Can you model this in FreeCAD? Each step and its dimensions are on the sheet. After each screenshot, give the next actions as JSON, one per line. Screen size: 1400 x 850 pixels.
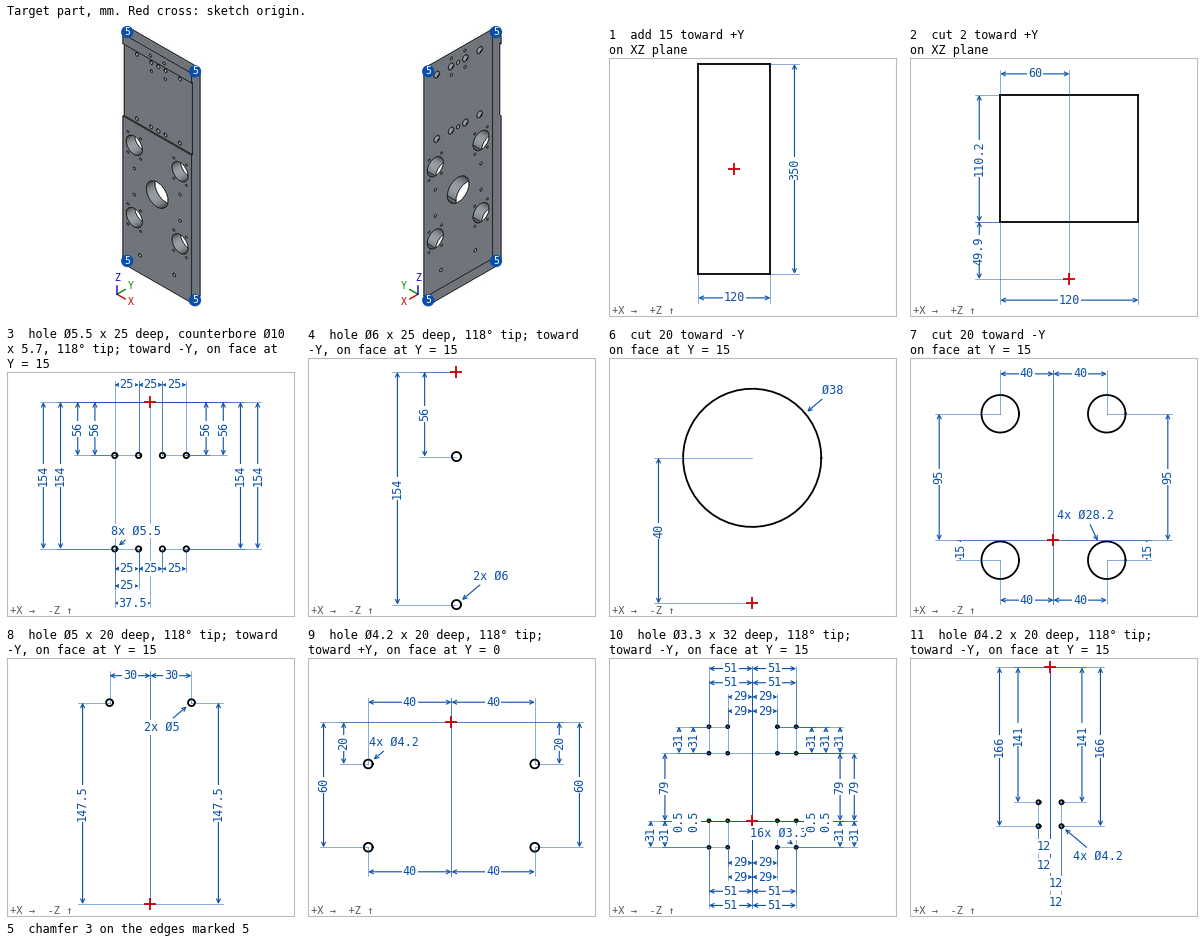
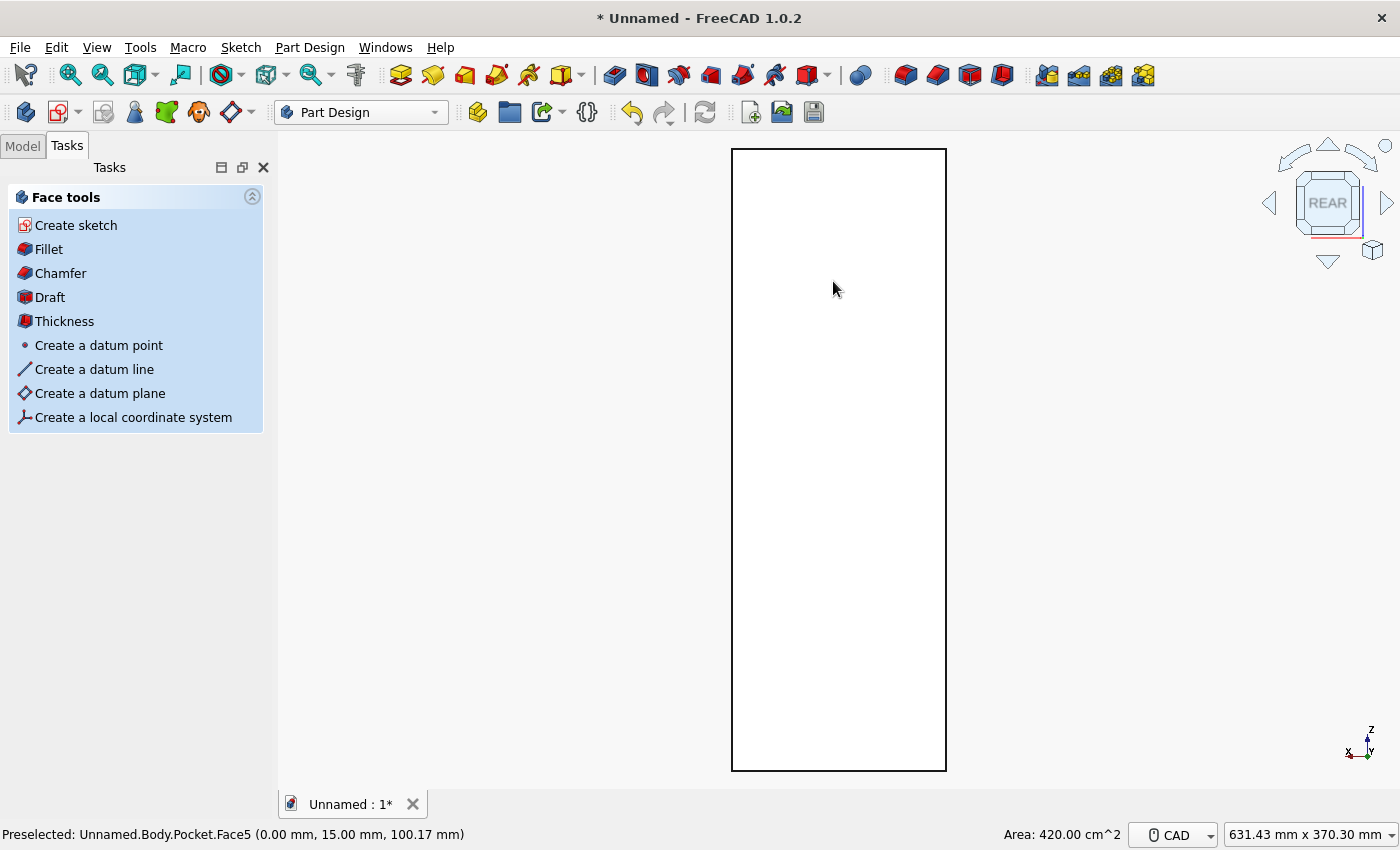
{"action": "left_click", "coordinate": [58, 112]}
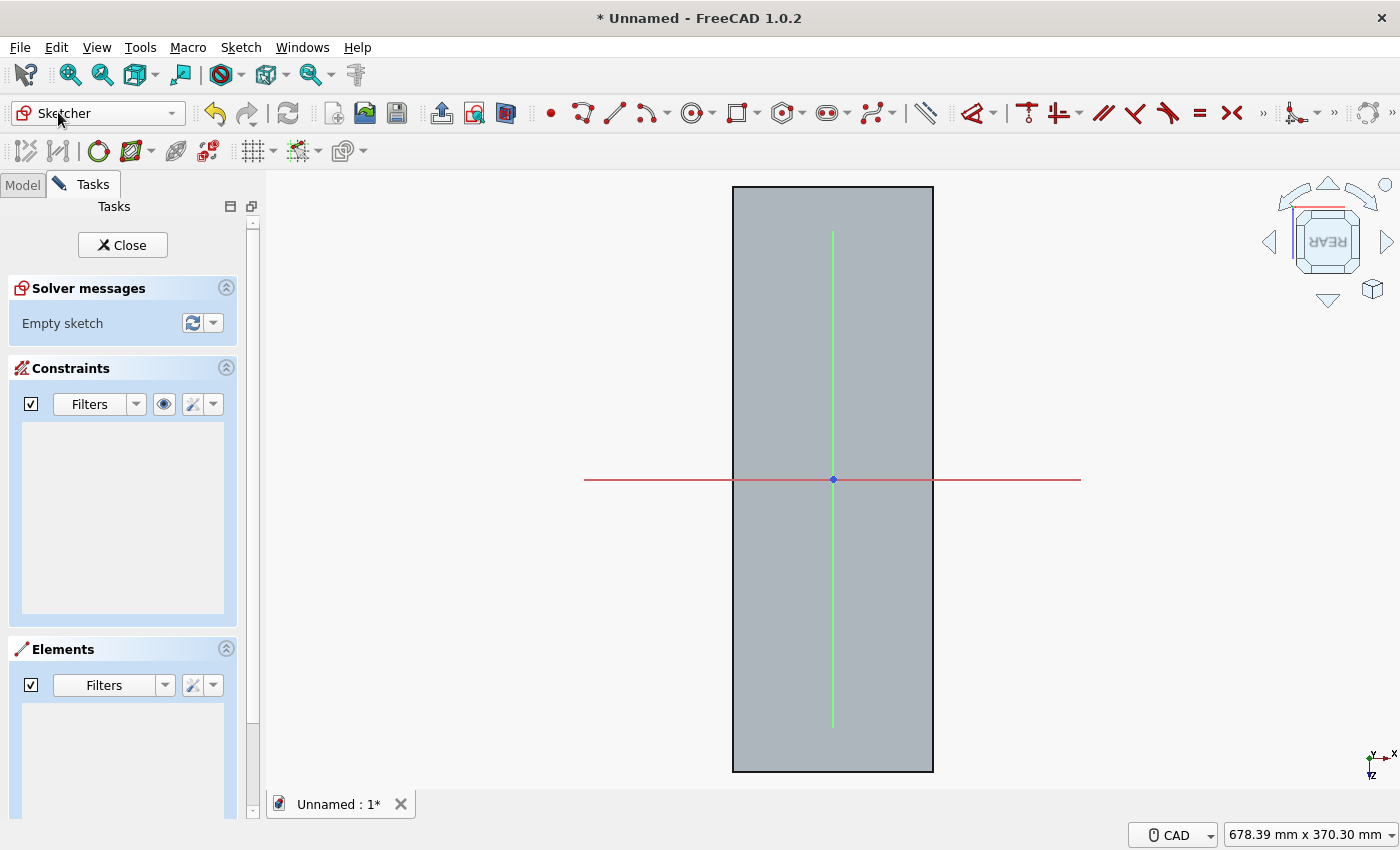
{"action": "scroll", "coordinate": [972, 761], "scroll_direction": "up", "scroll_amount": 2}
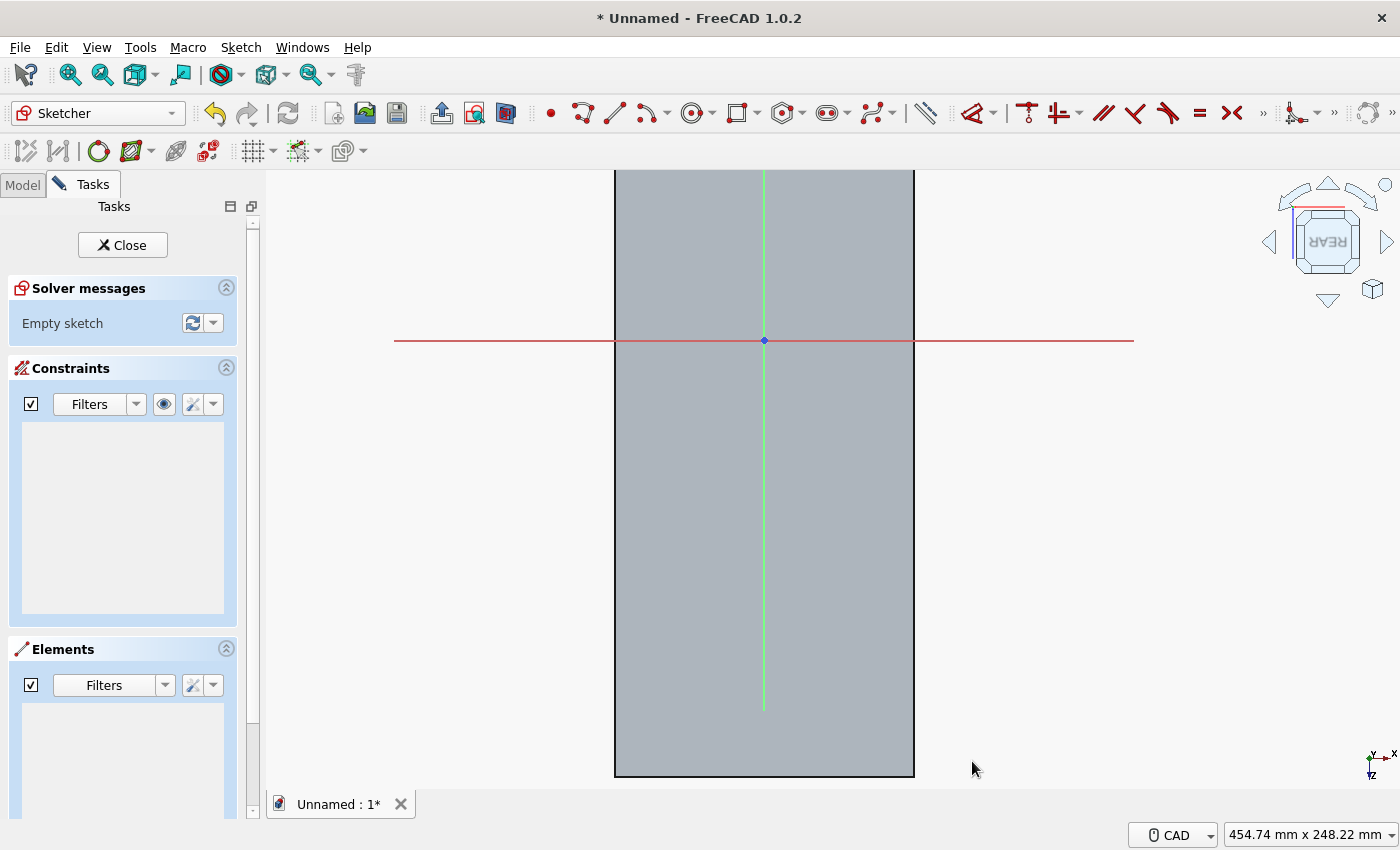
{"action": "left_click", "coordinate": [692, 114]}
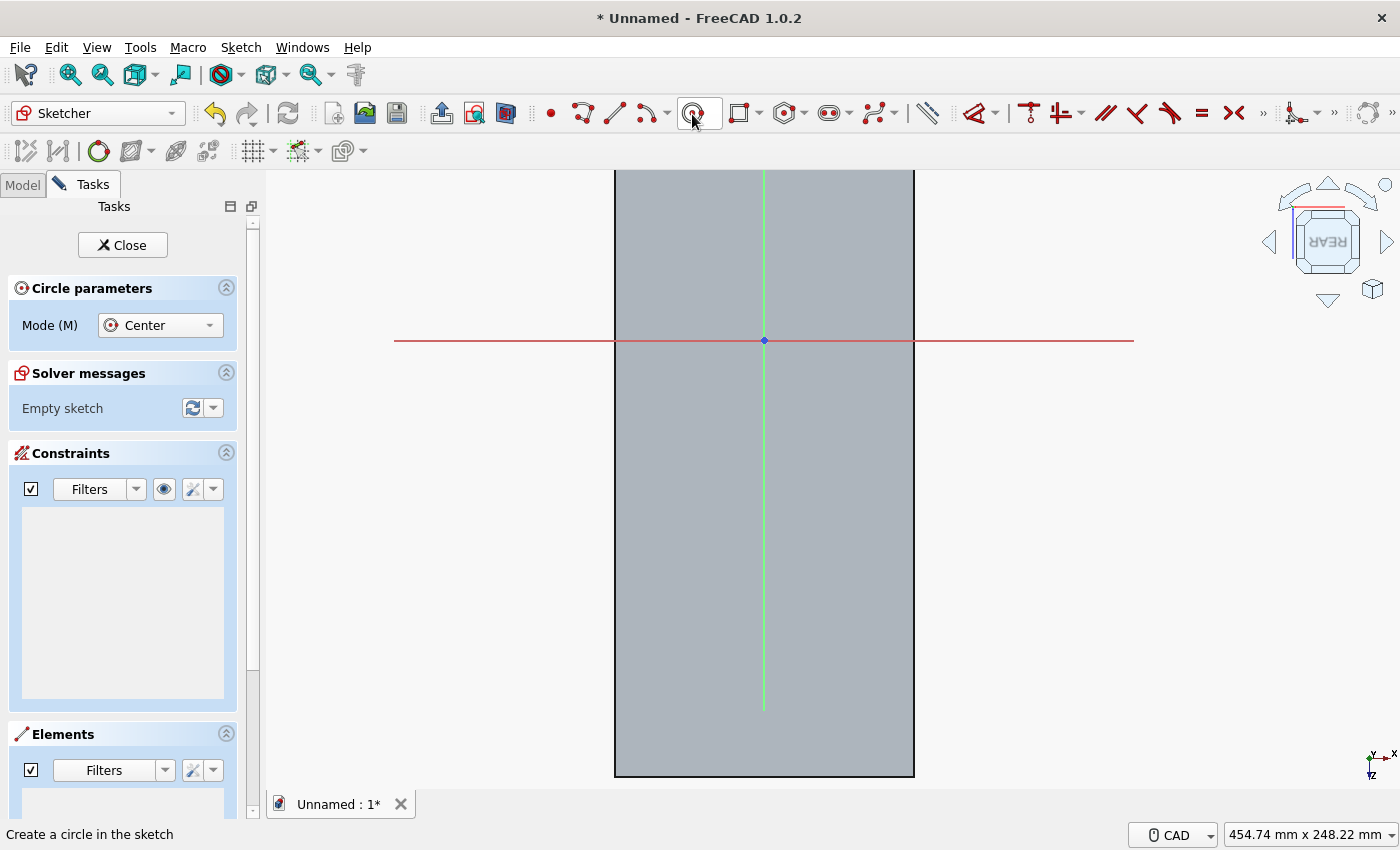
{"action": "scroll", "coordinate": [671, 725], "scroll_direction": "up", "scroll_amount": 6}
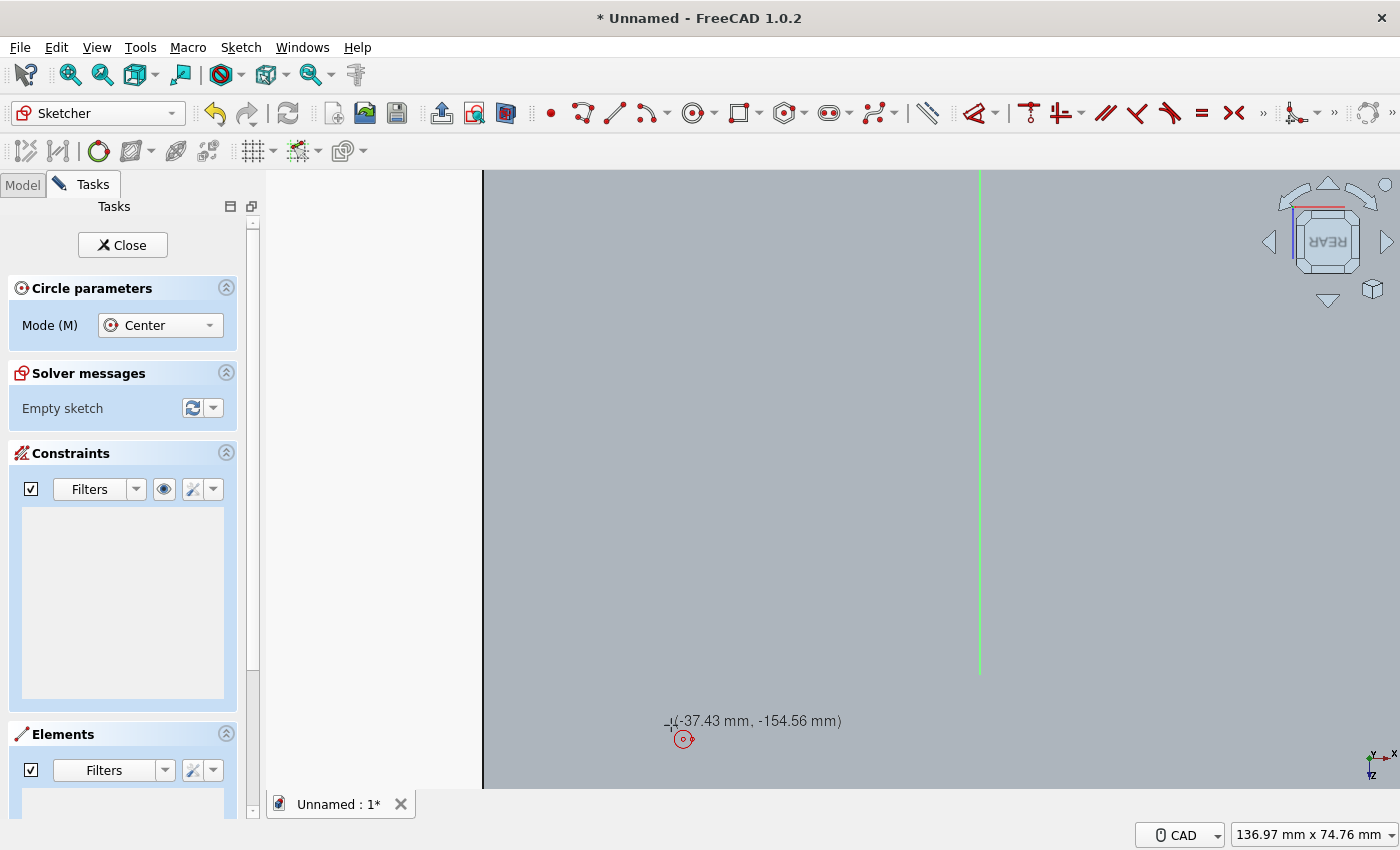
{"action": "left_click", "coordinate": [670, 722]}
{"action": "left_click", "coordinate": [686, 706]}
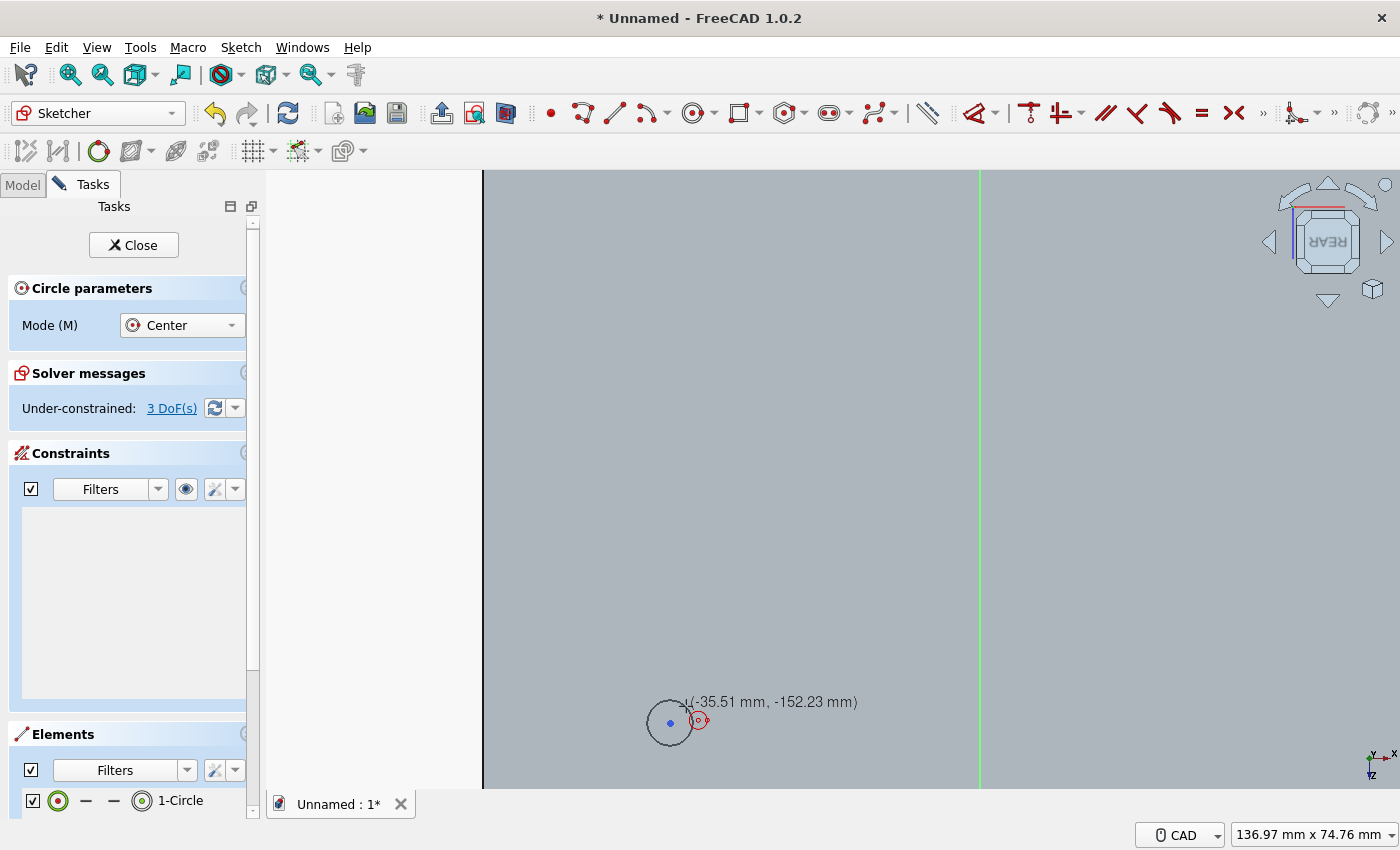
{"action": "left_click", "coordinate": [877, 722]}
{"action": "left_click", "coordinate": [893, 706]}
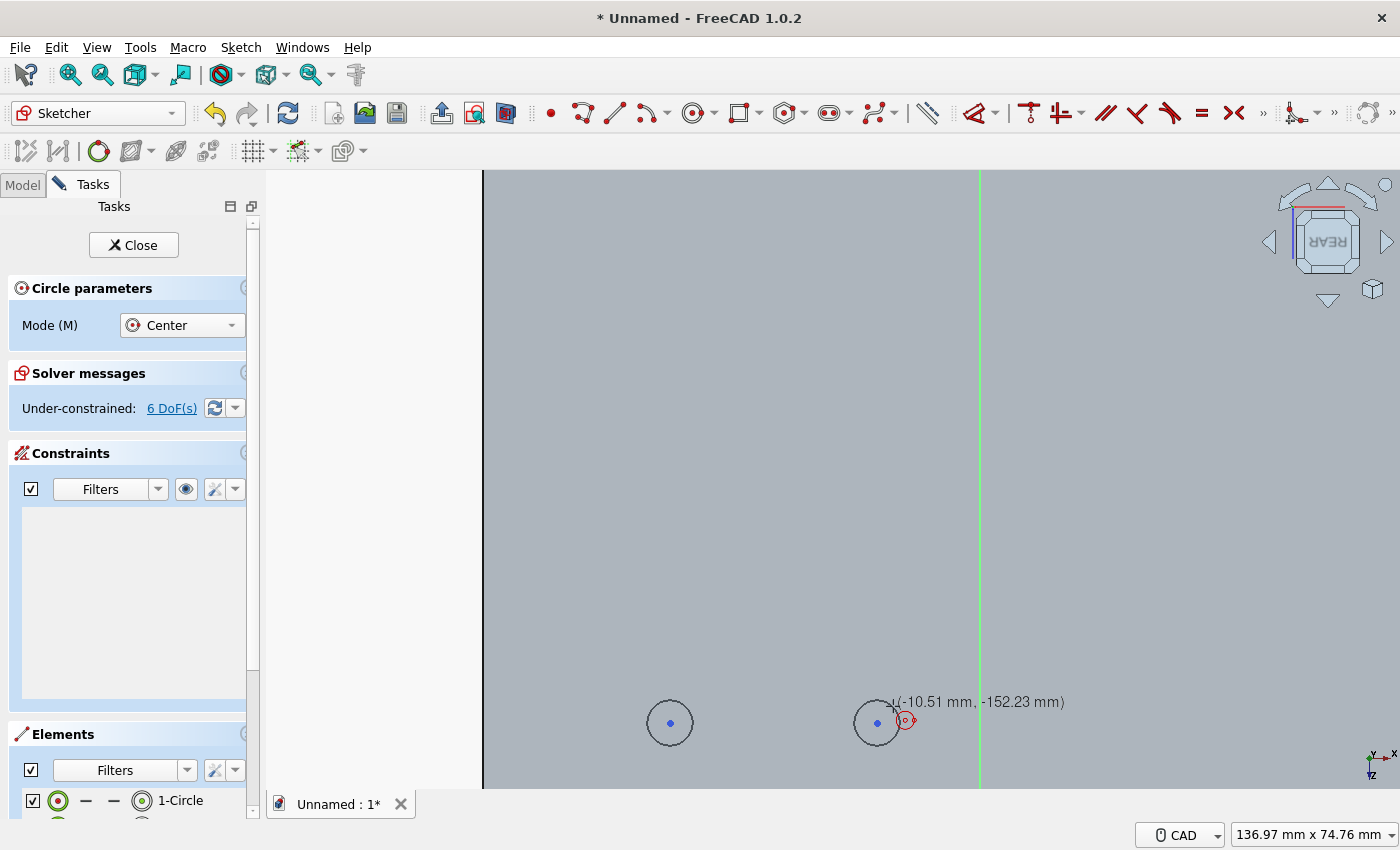
{"action": "left_click", "coordinate": [1084, 722]}
{"action": "left_click", "coordinate": [1100, 706]}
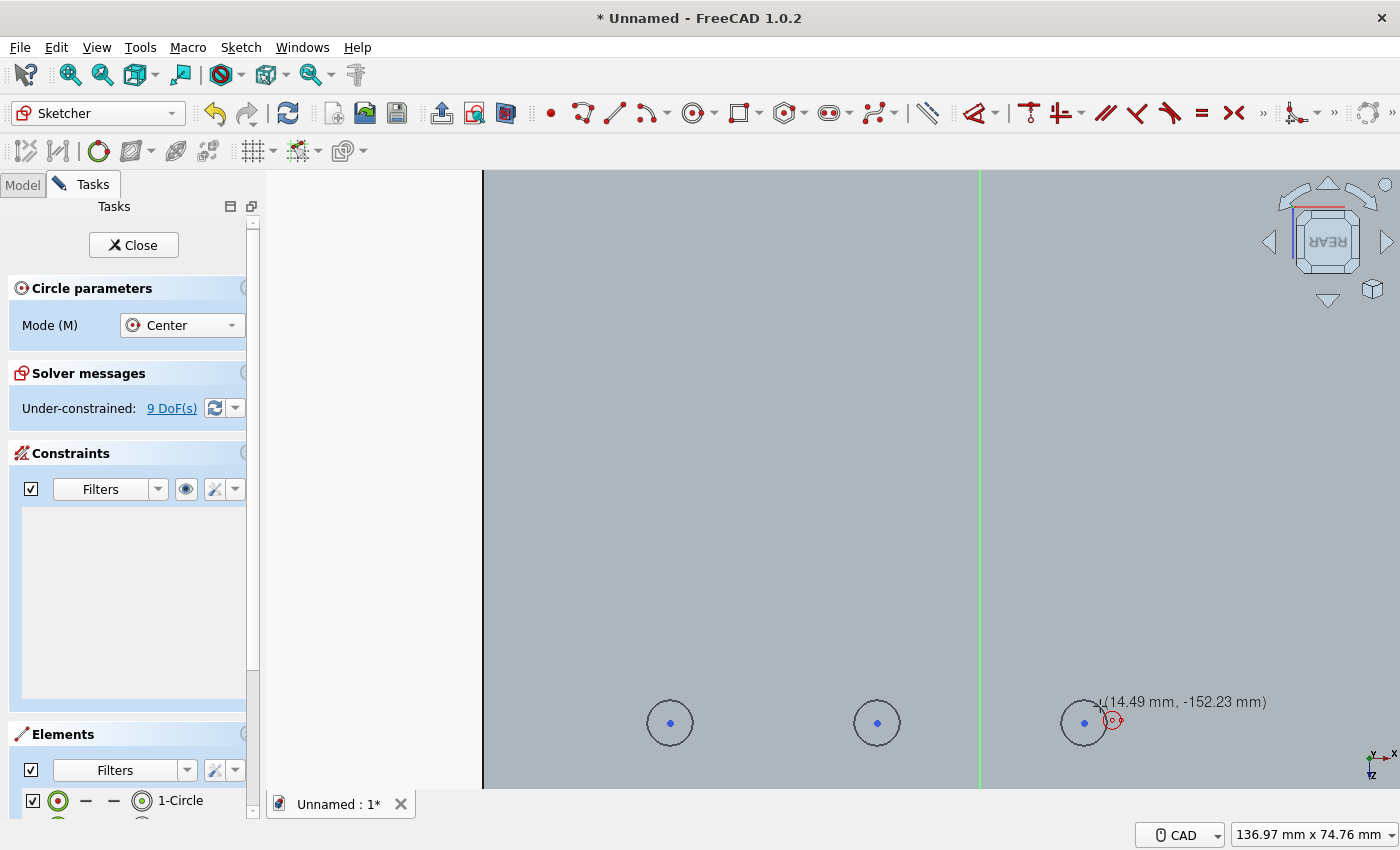
{"action": "scroll", "coordinate": [672, 645], "scroll_direction": "down", "scroll_amount": 6}